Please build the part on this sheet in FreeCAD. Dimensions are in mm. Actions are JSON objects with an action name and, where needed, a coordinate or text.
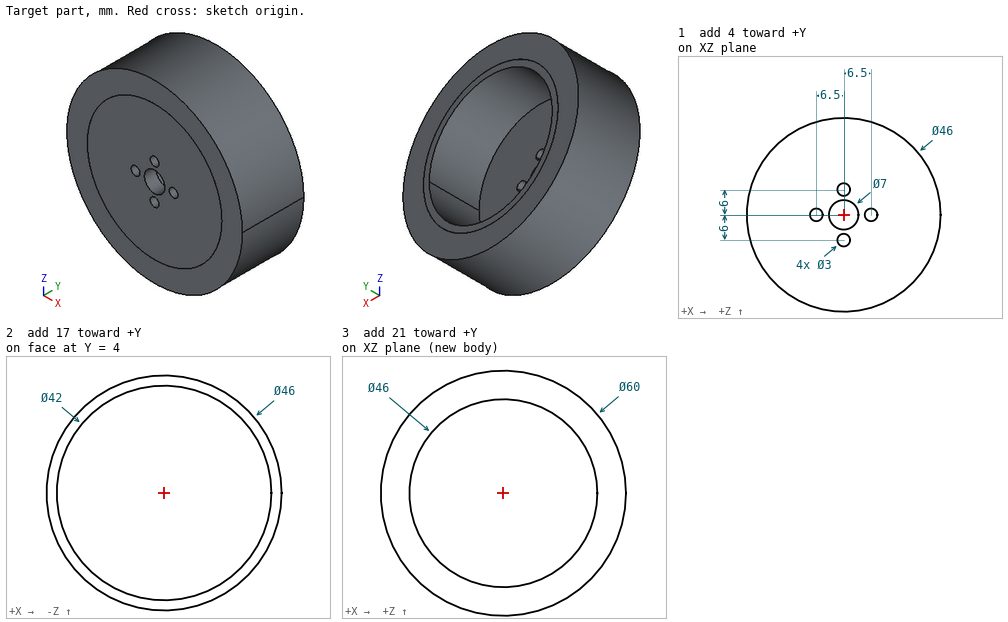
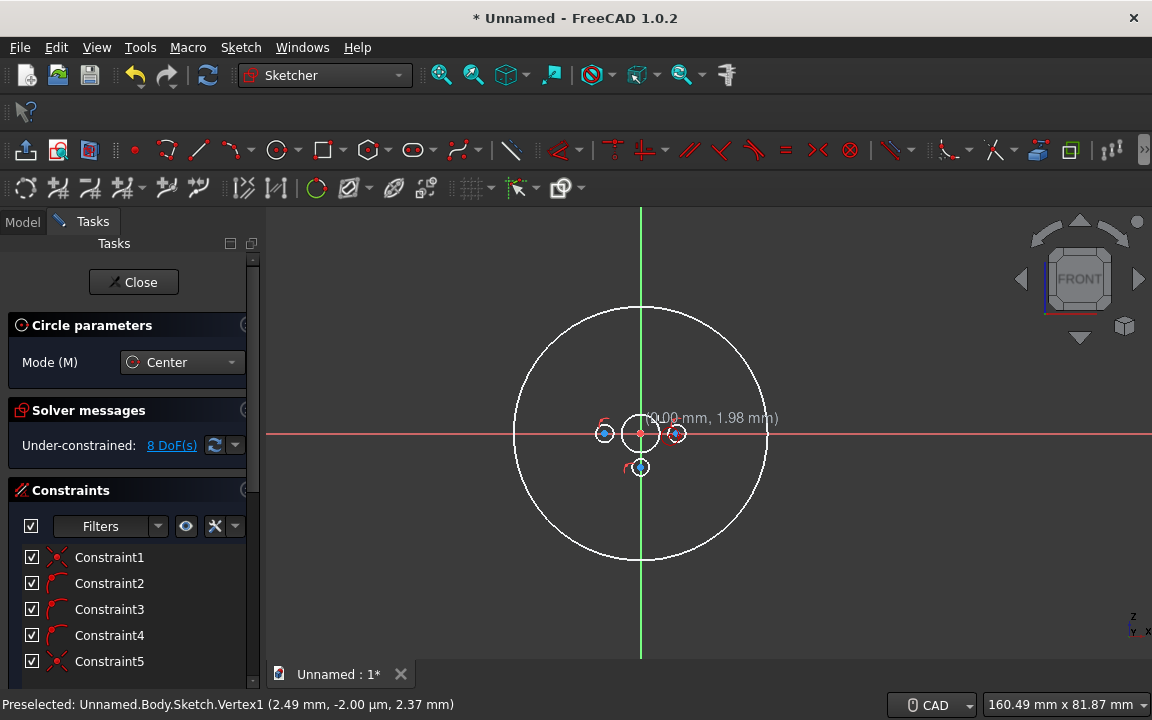
{"action": "left_click", "coordinate": [641, 400]}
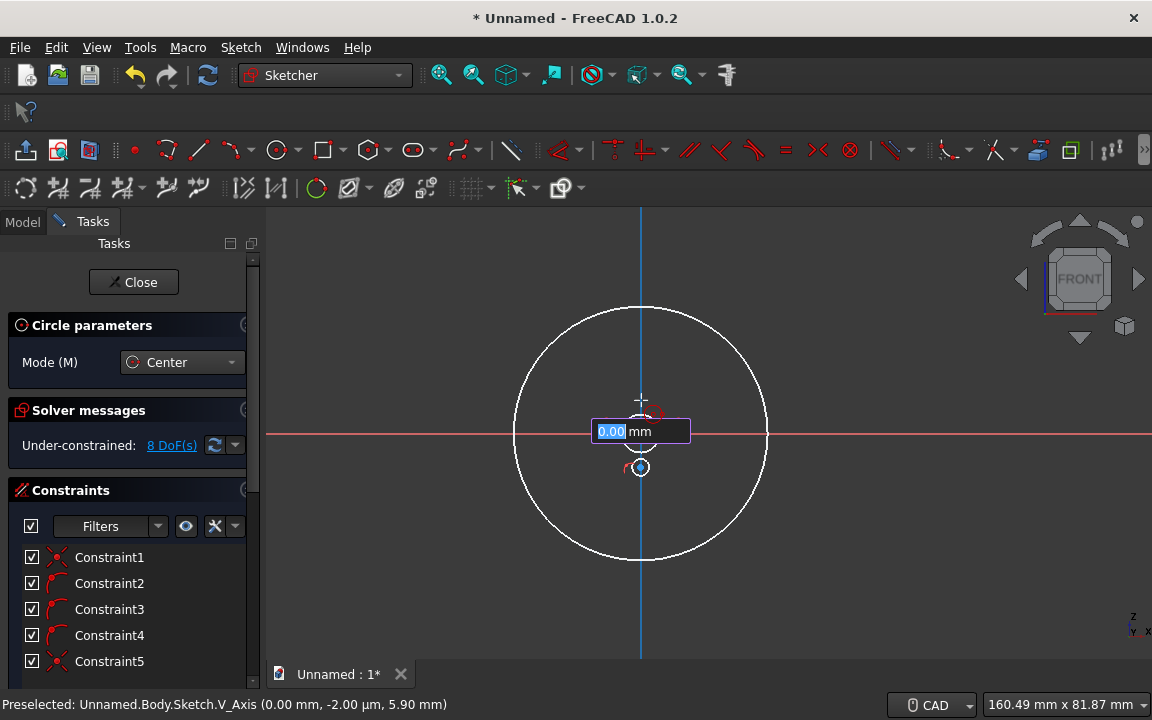
{"action": "scroll", "coordinate": [648, 398], "scroll_direction": "up", "scroll_amount": 4}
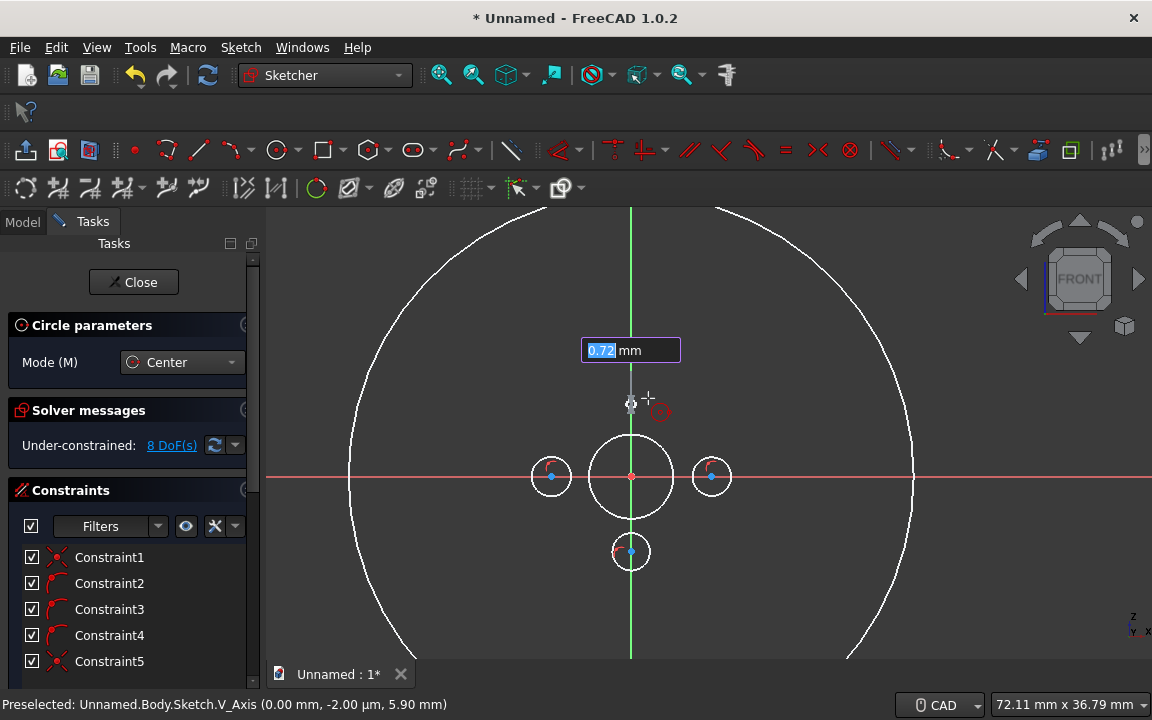
{"action": "left_click", "coordinate": [648, 397]}
{"action": "key", "text": "Escape"}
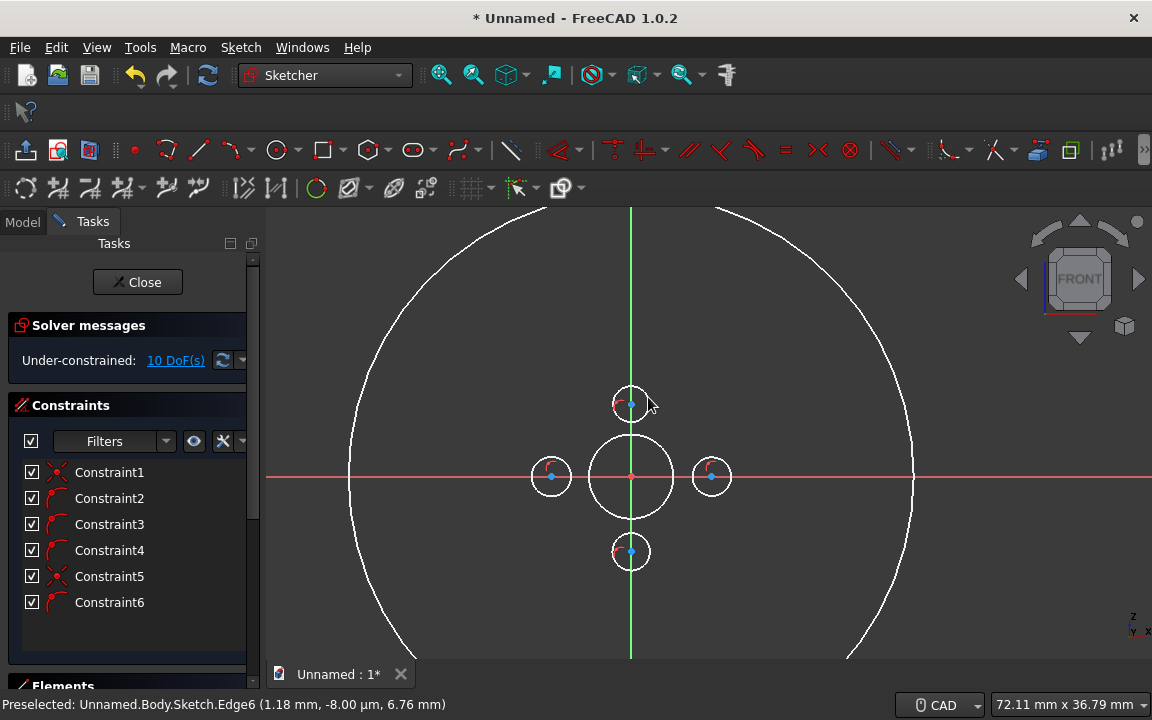
{"action": "left_click", "coordinate": [644, 539]}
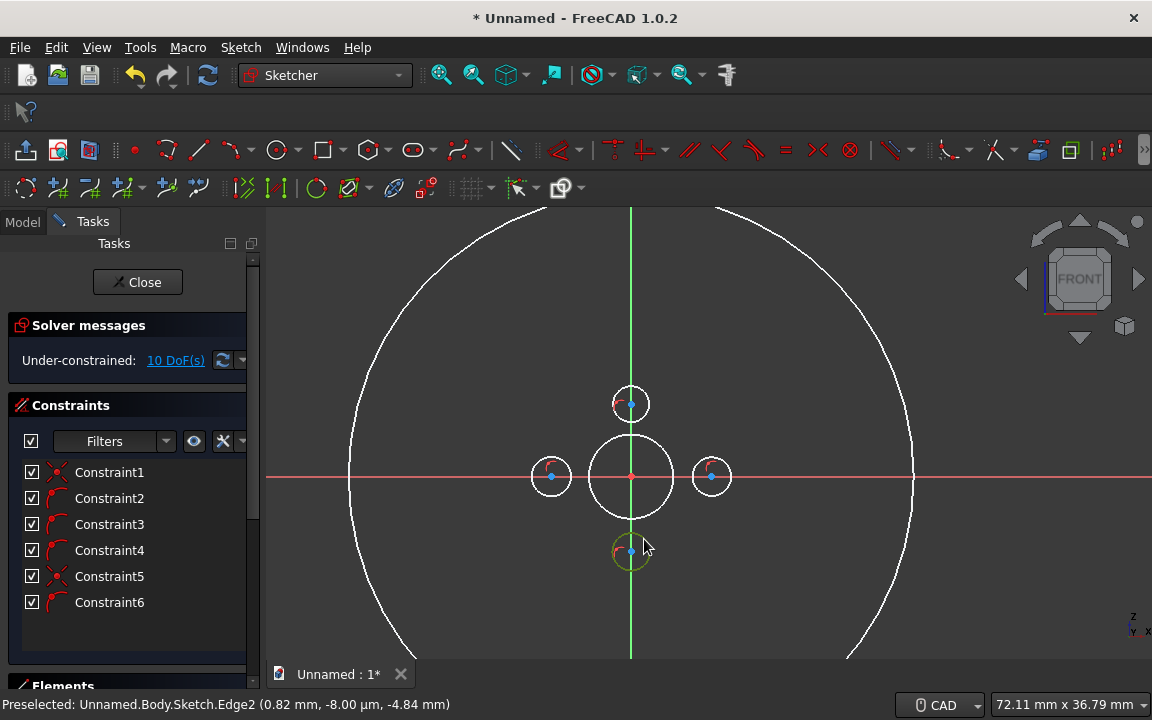
{"action": "left_click", "coordinate": [565, 463]}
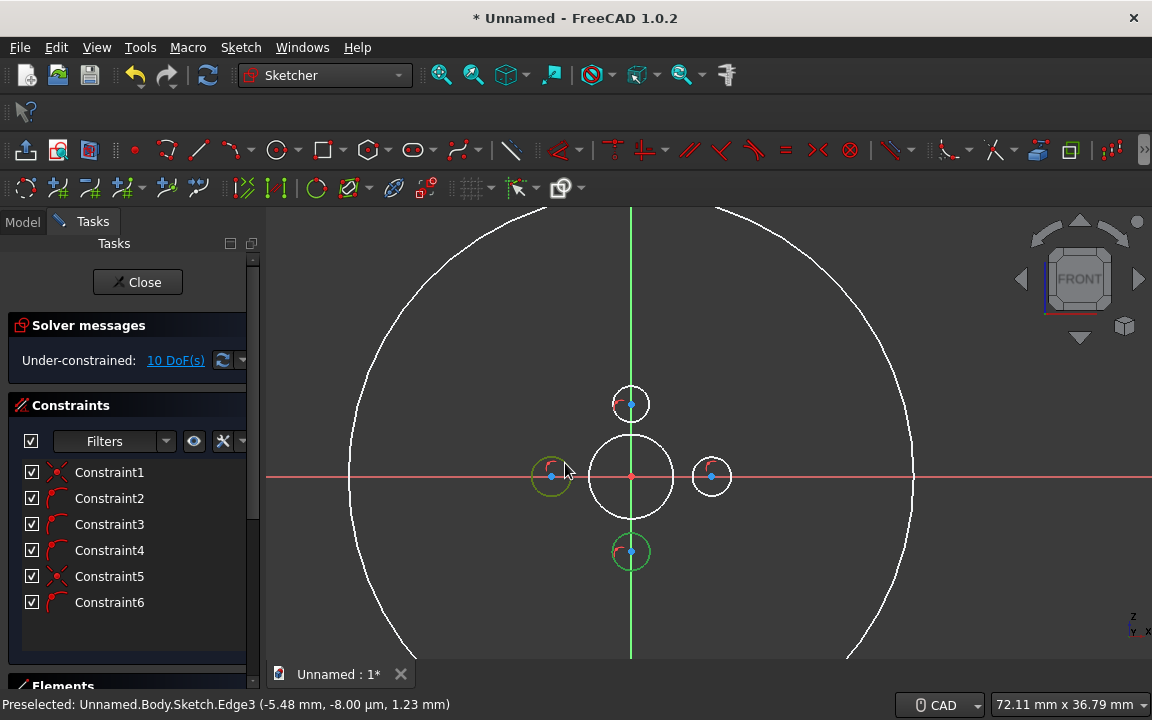
{"action": "left_click", "coordinate": [725, 463]}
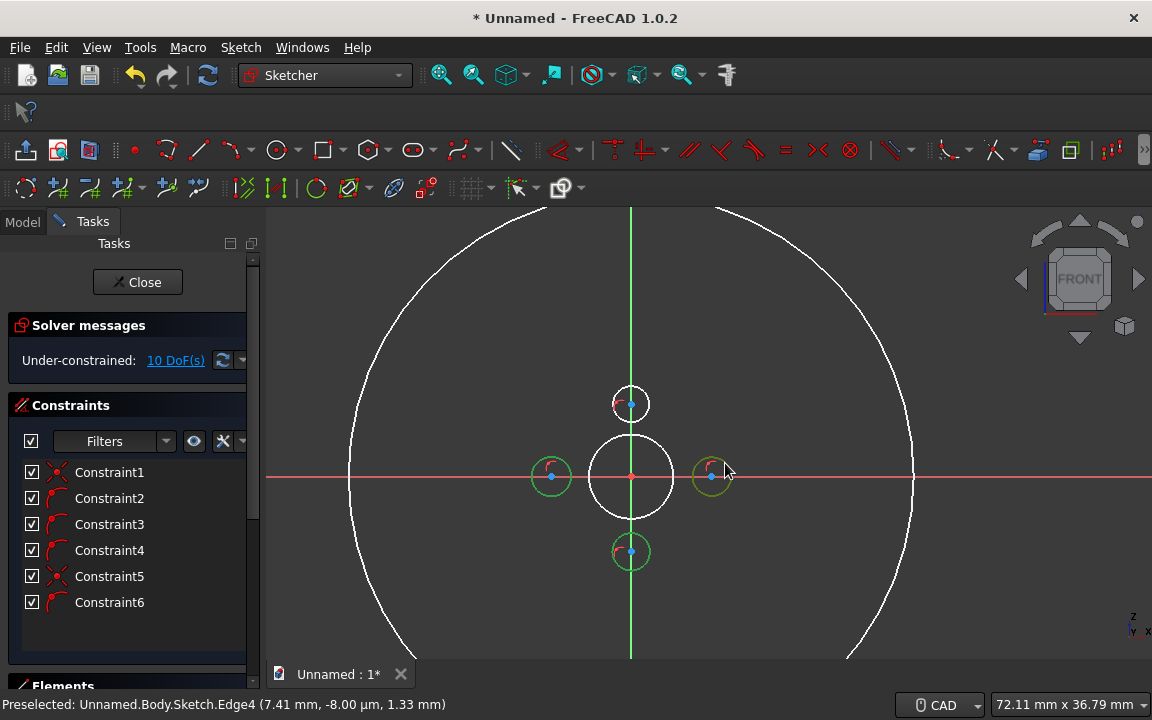
{"action": "left_click", "coordinate": [644, 391]}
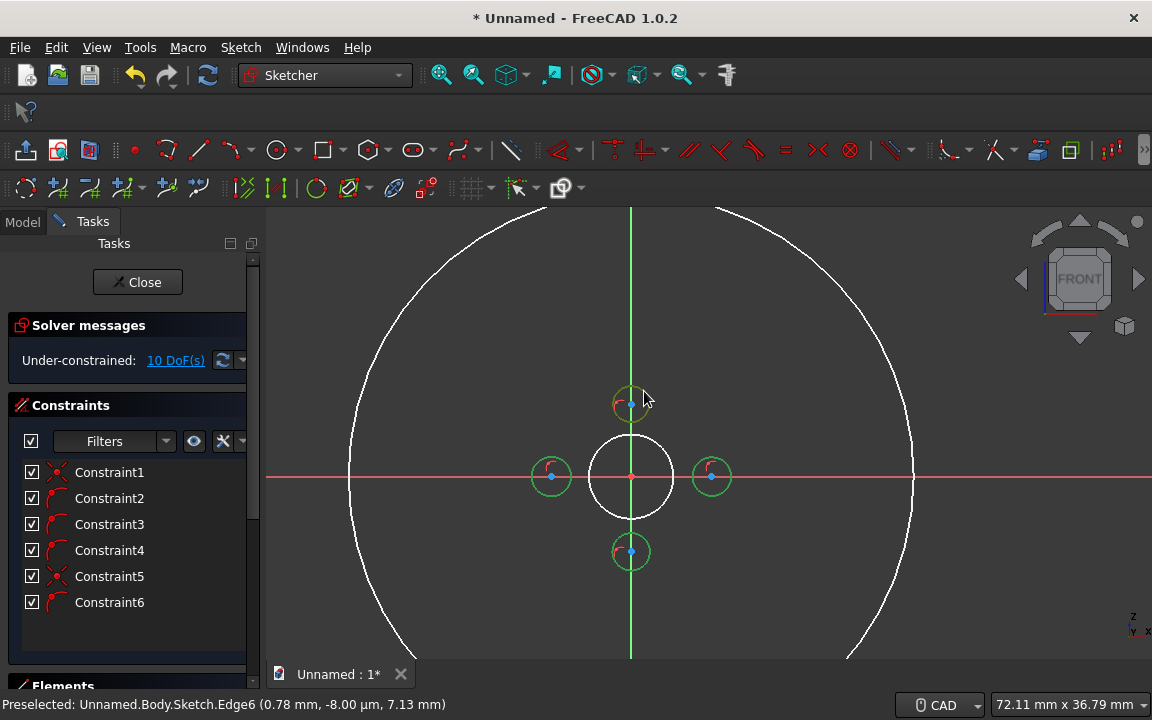
{"action": "left_click", "coordinate": [786, 150]}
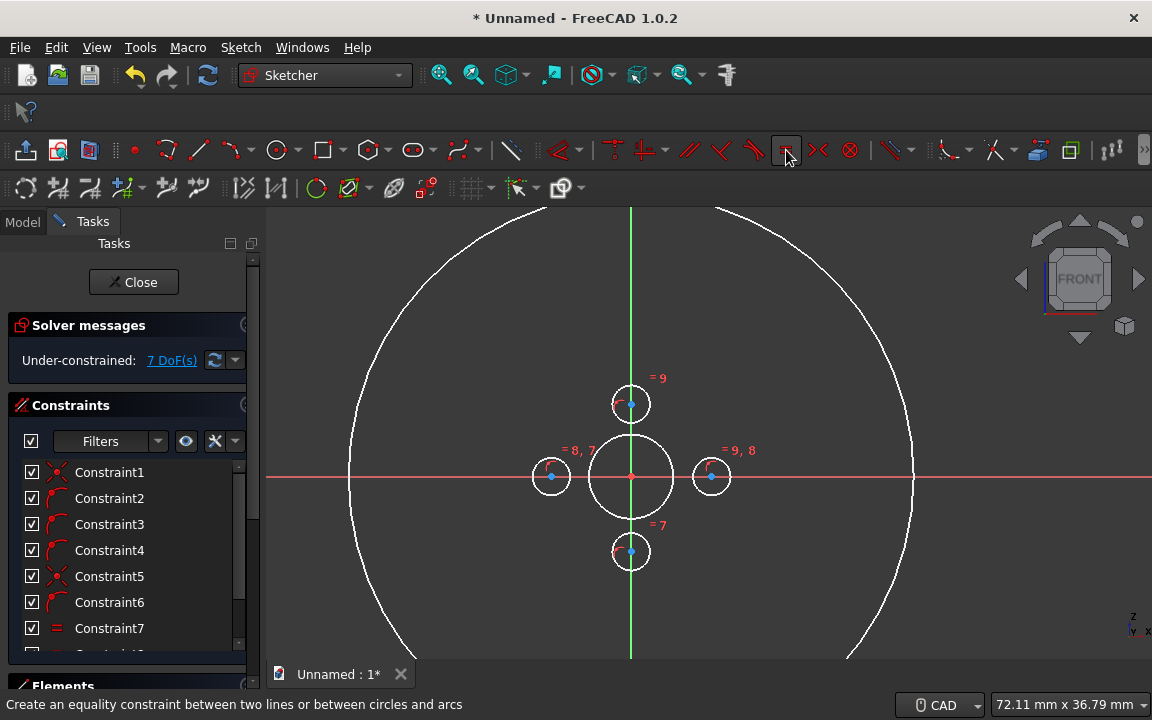
{"action": "left_click", "coordinate": [830, 276]}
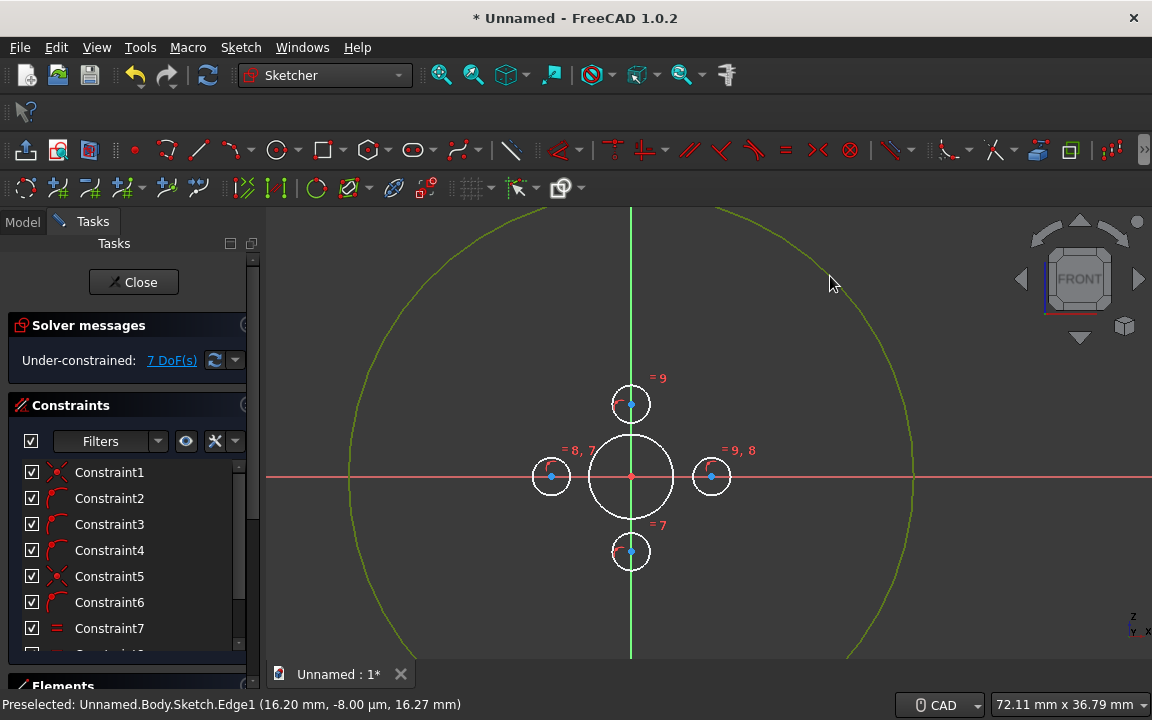
{"action": "key", "text": "k o"}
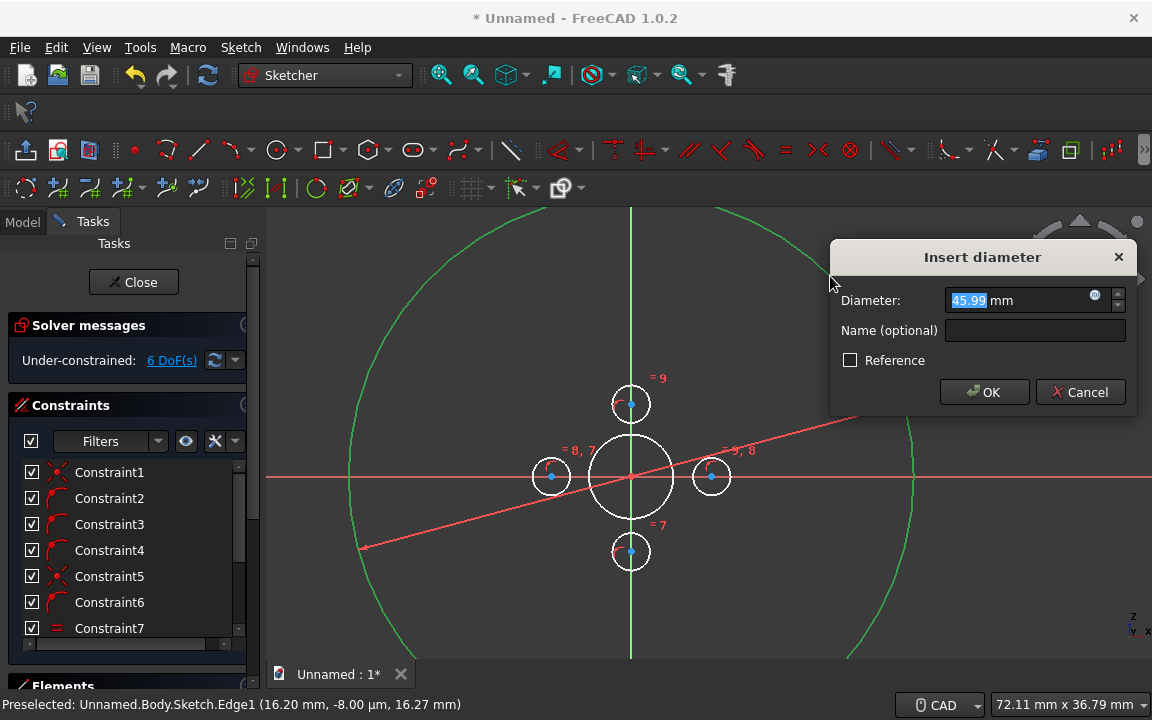
{"action": "type", "text": "46"}
{"action": "key", "text": "Return"}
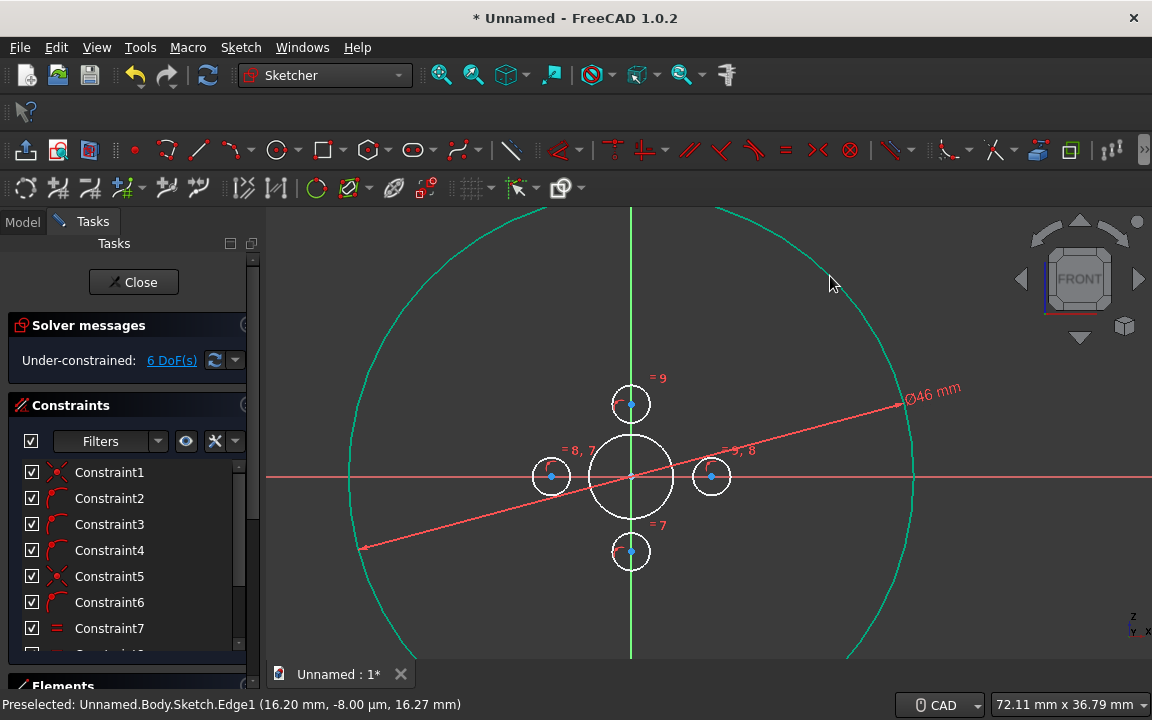
{"action": "left_click", "coordinate": [644, 539]}